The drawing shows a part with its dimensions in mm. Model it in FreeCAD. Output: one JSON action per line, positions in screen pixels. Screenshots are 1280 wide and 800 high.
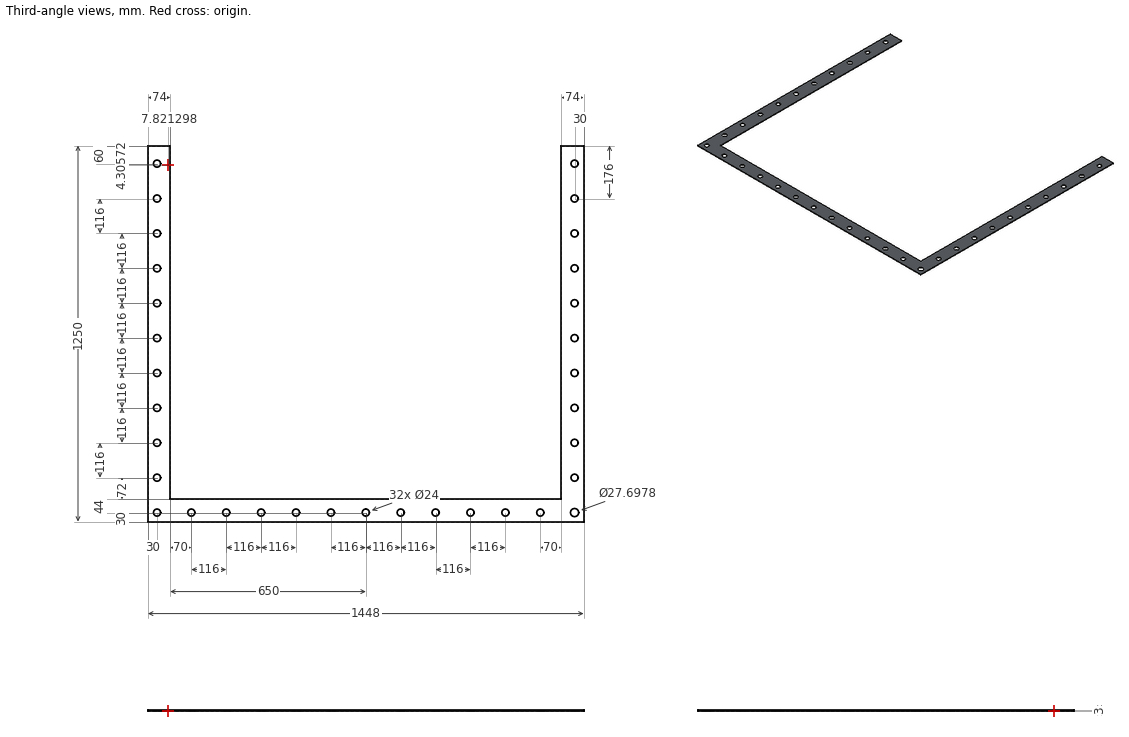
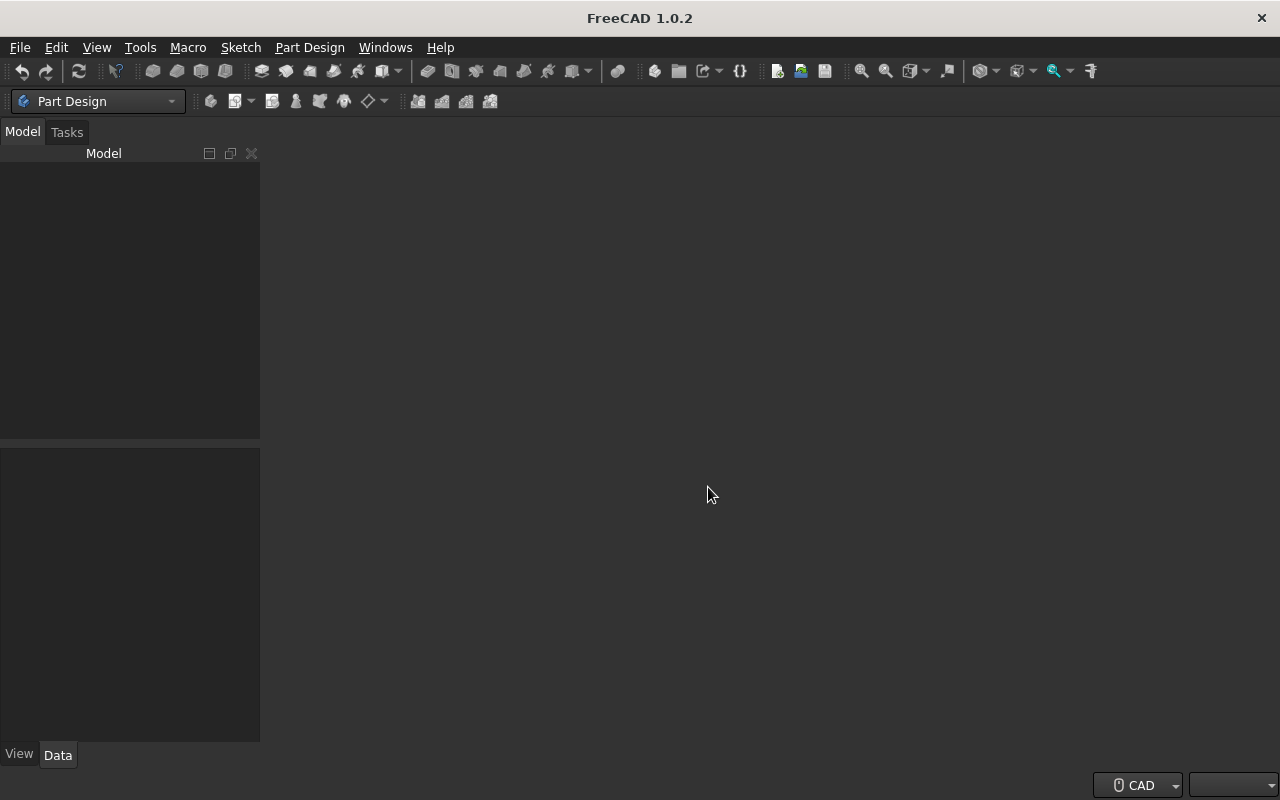
{"action": "left_click", "coordinate": [778, 72]}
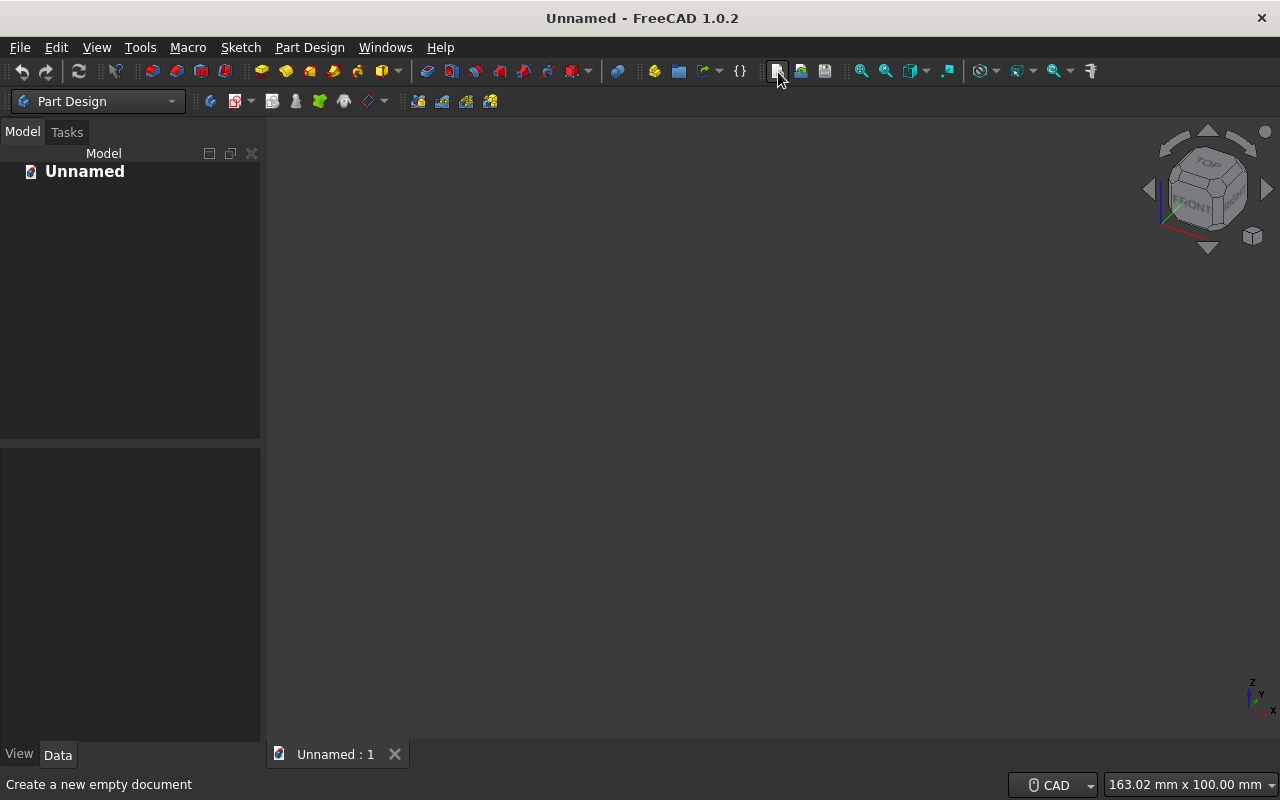
{"action": "left_click", "coordinate": [236, 102]}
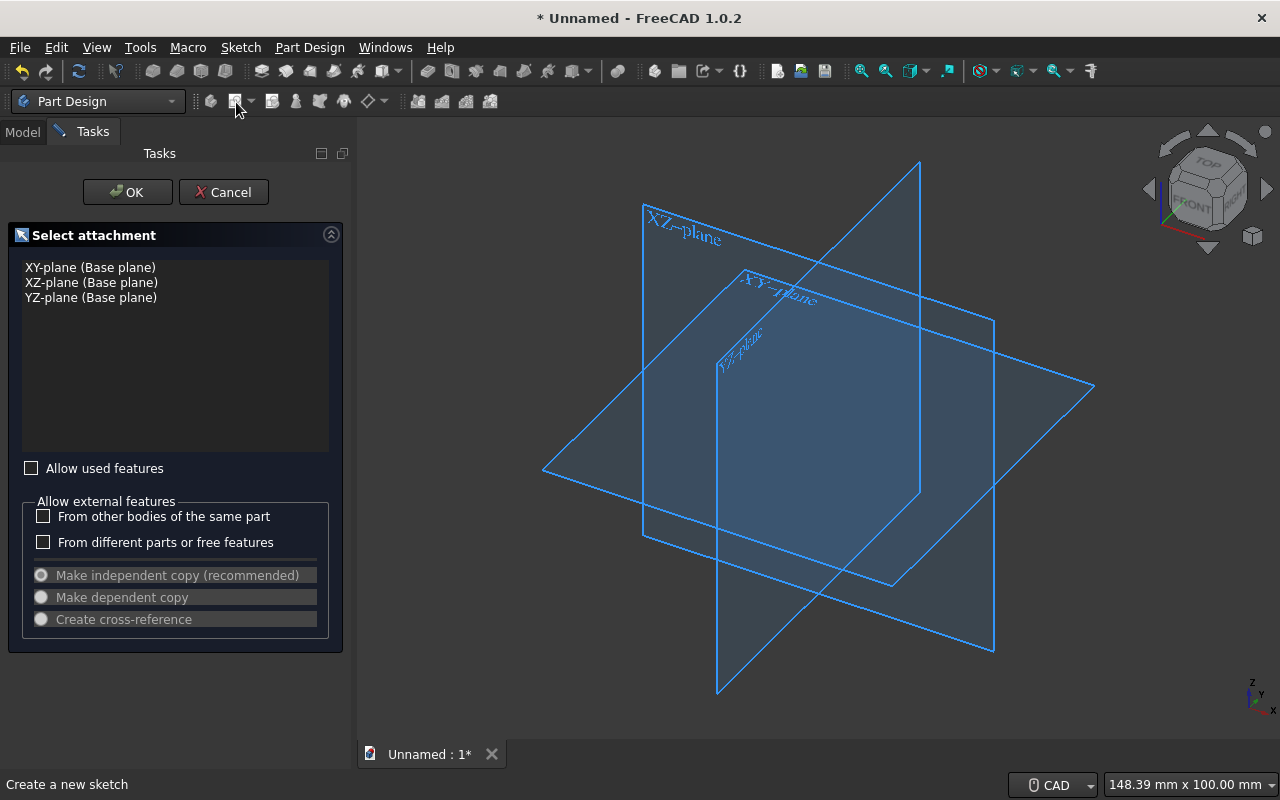
{"action": "left_click", "coordinate": [82, 268]}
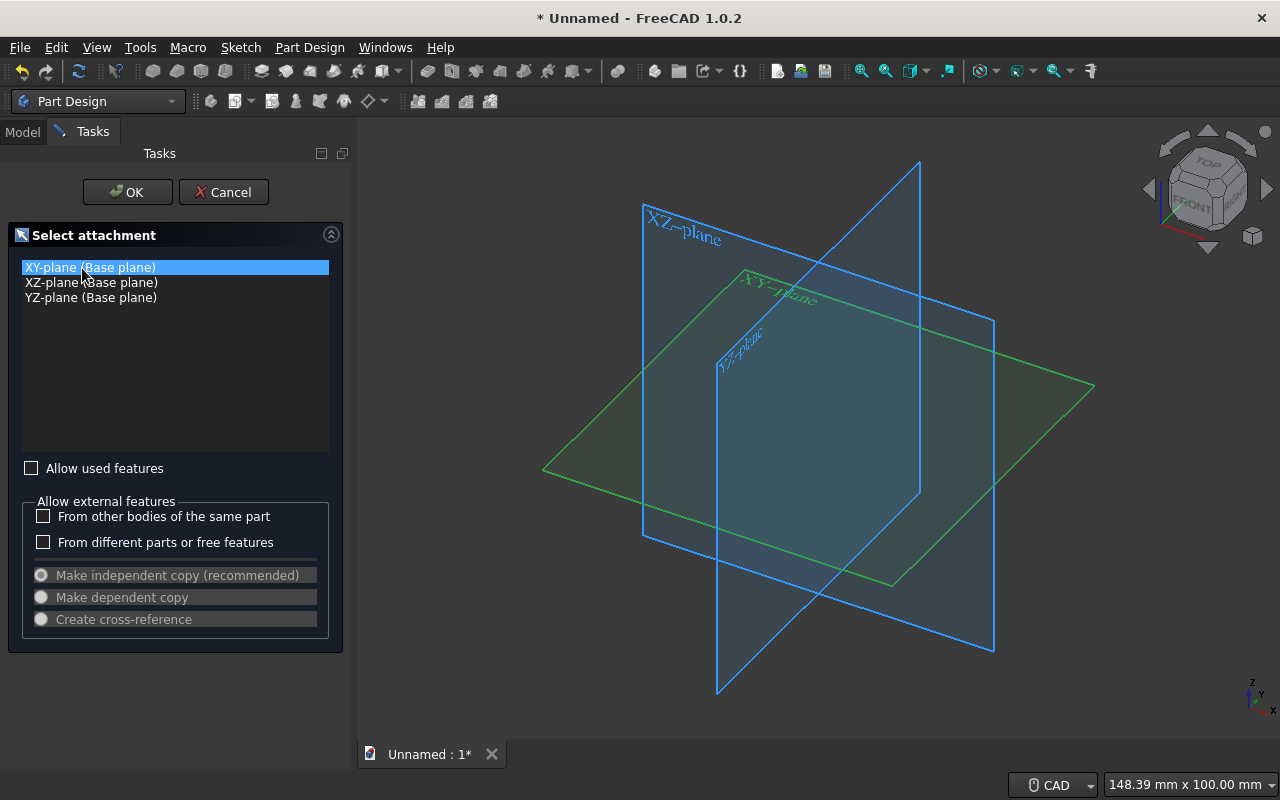
{"action": "left_click", "coordinate": [128, 192]}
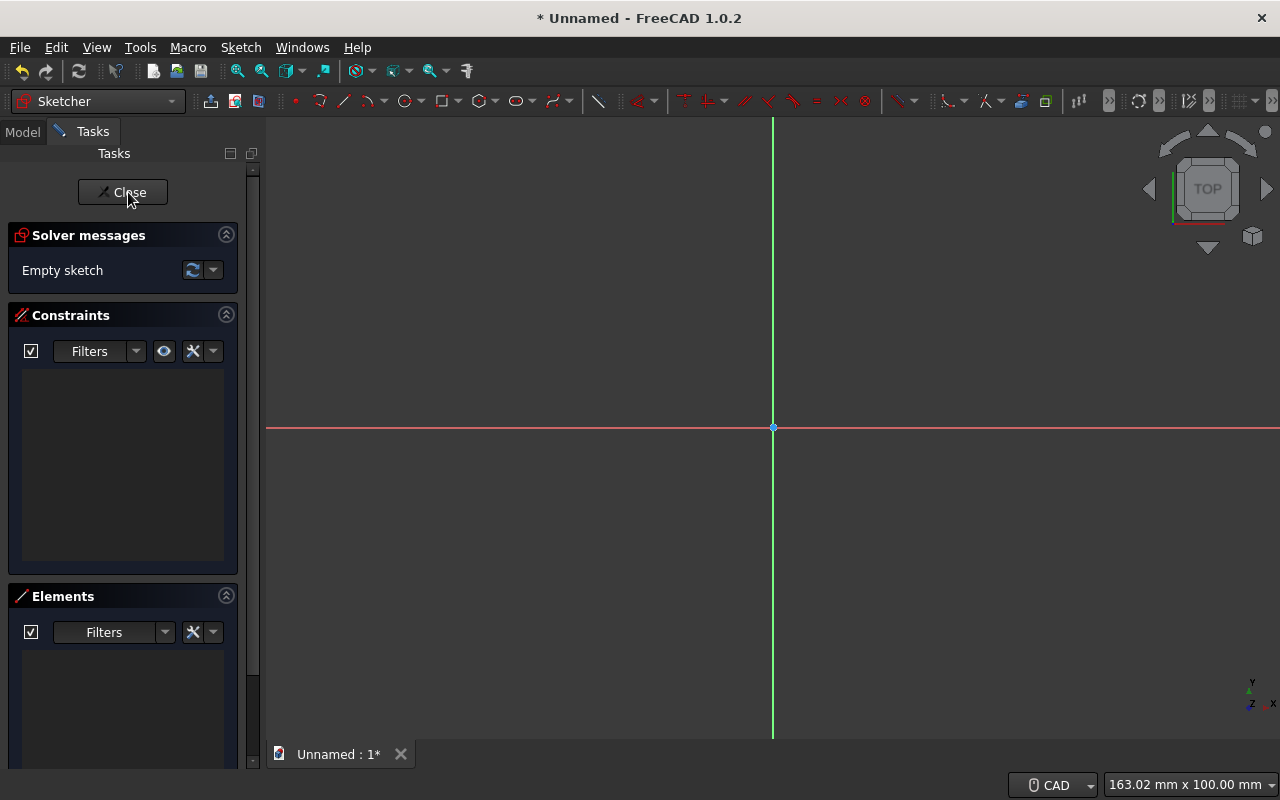
{"action": "scroll", "coordinate": [487, 245], "scroll_direction": "down", "scroll_amount": 15}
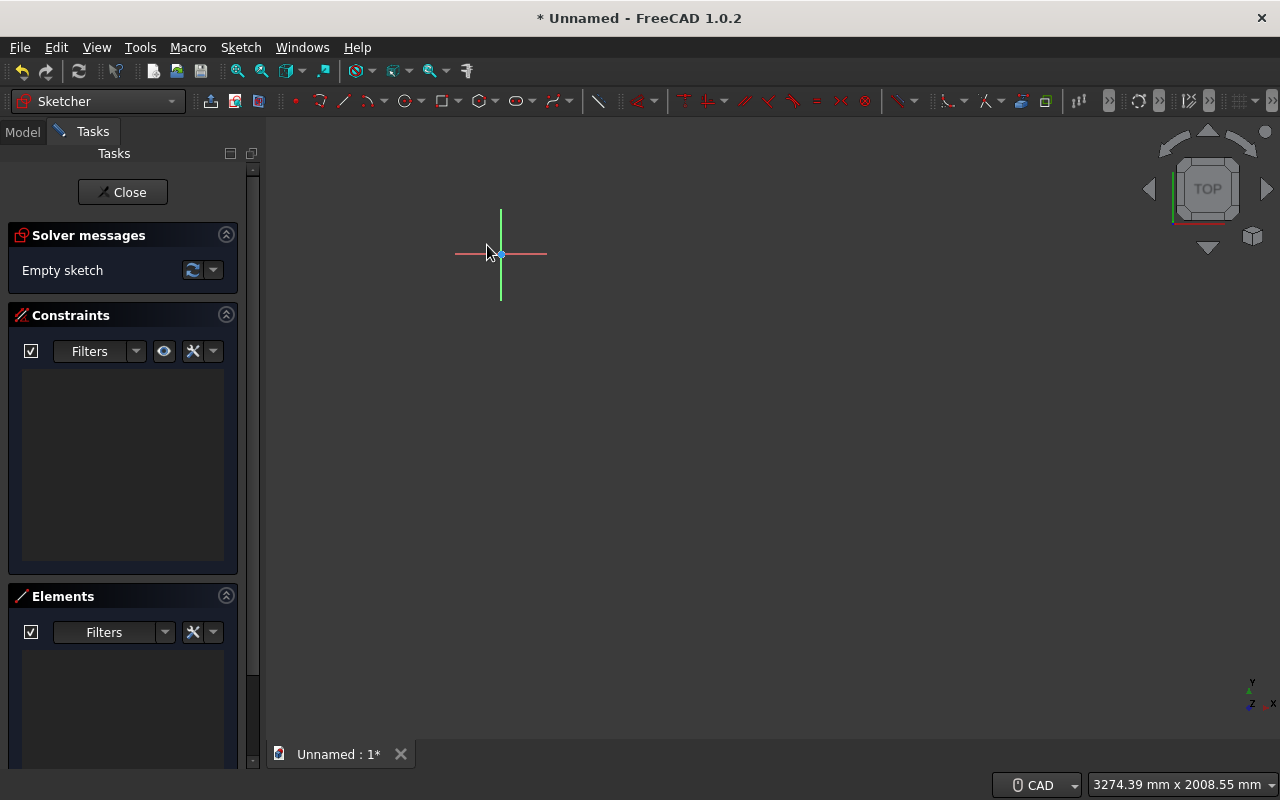
{"action": "left_click", "coordinate": [320, 102]}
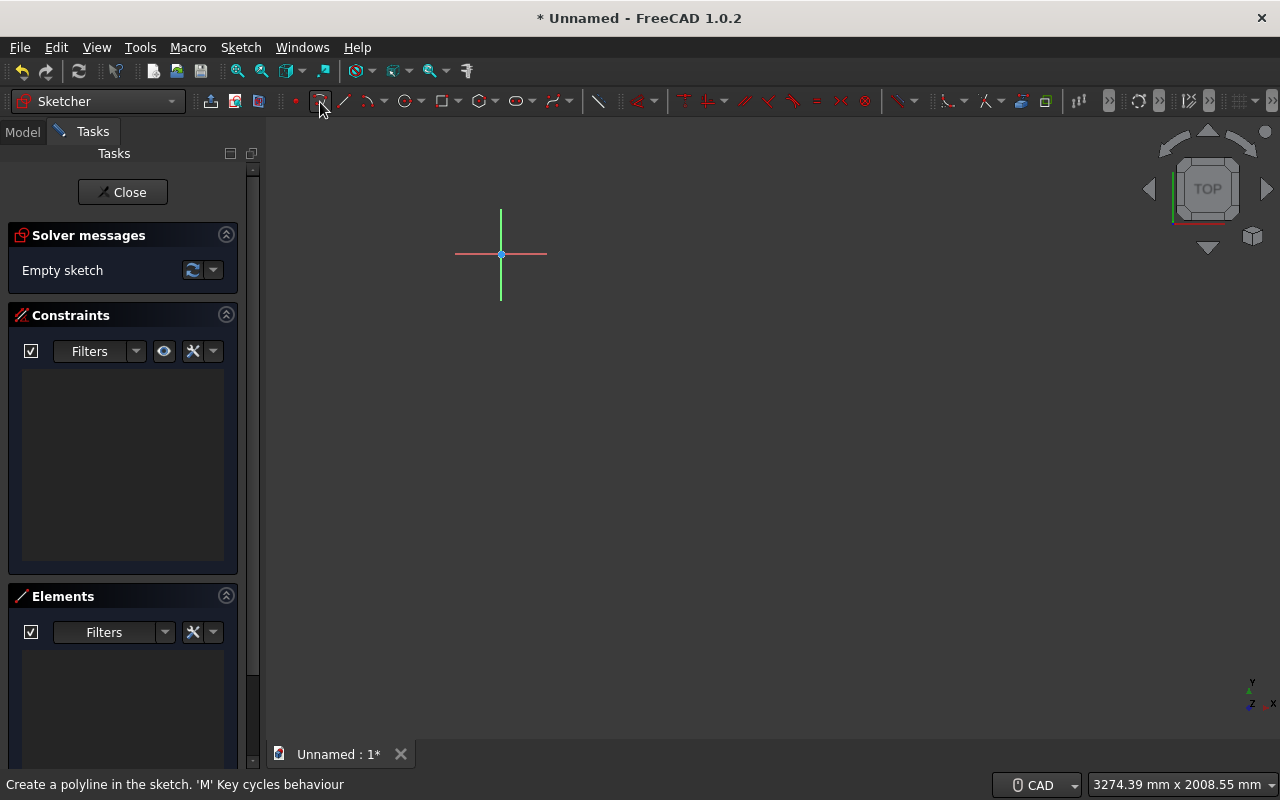
{"action": "scroll", "coordinate": [504, 234], "scroll_direction": "up", "scroll_amount": 10}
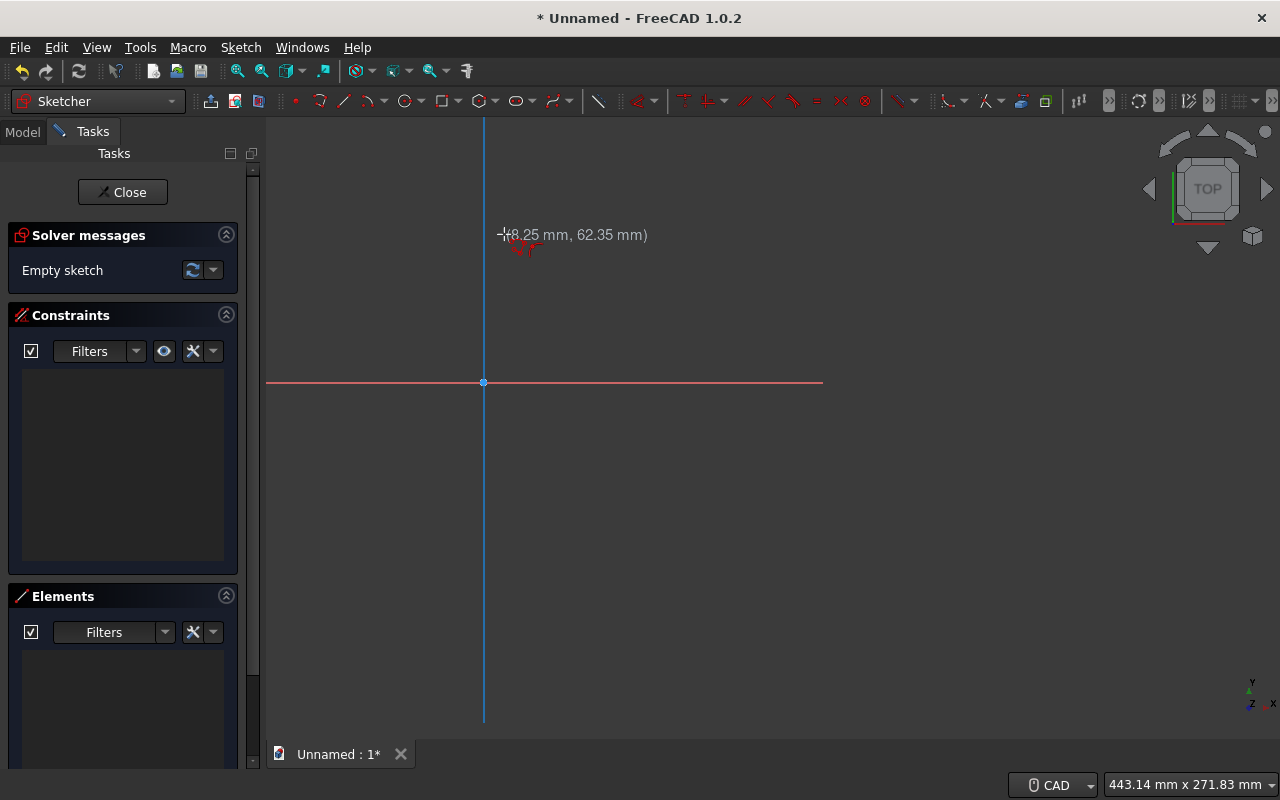
{"action": "left_click", "coordinate": [502, 236]}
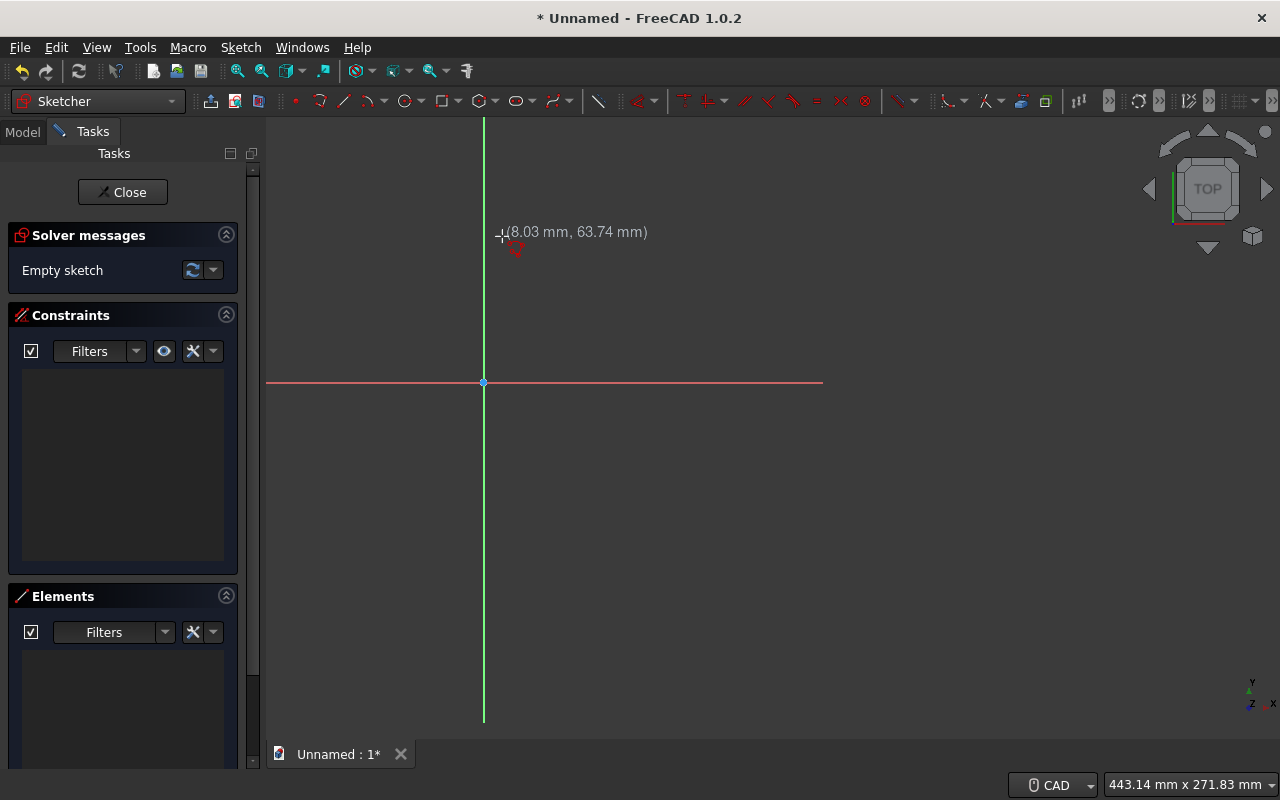
{"action": "scroll", "coordinate": [503, 234], "scroll_direction": "down", "scroll_amount": 10}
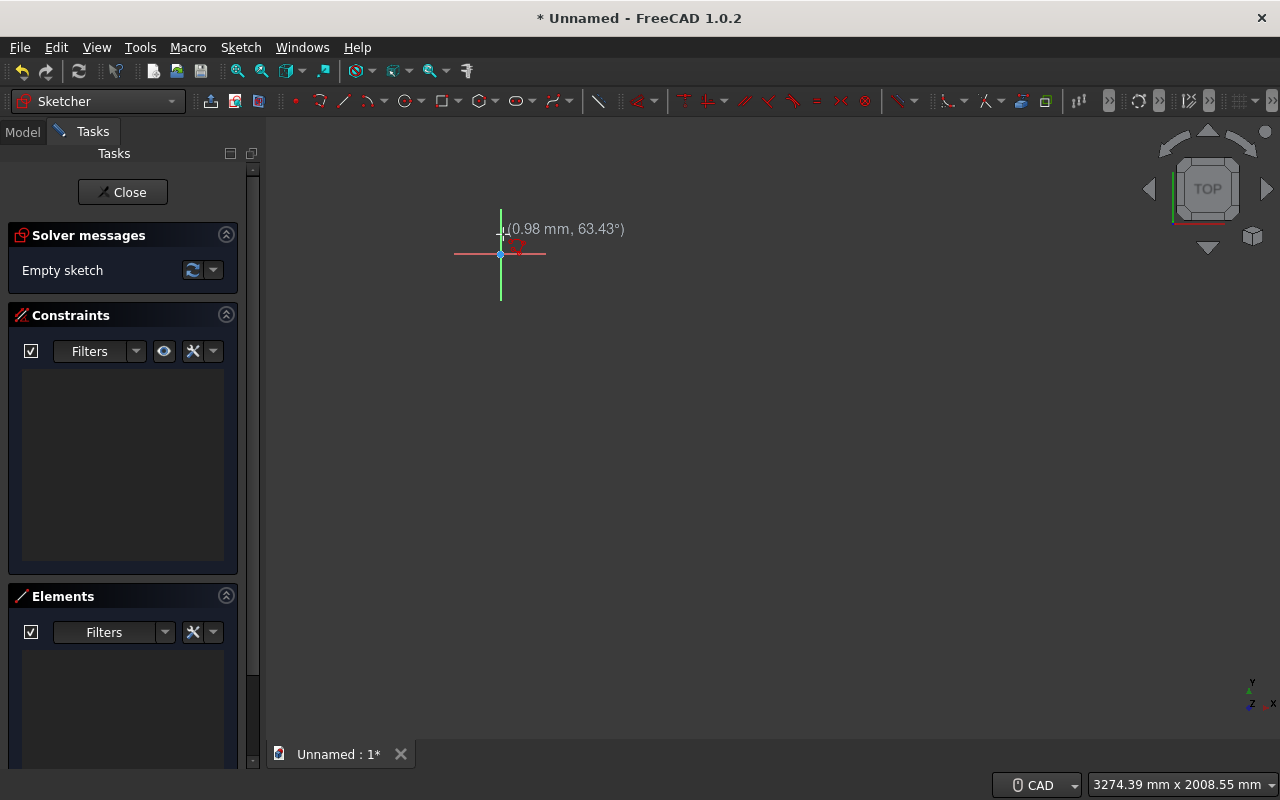
{"action": "left_click", "coordinate": [480, 234]}
{"action": "left_click", "coordinate": [480, 621]}
{"action": "left_click", "coordinate": [928, 621]}
{"action": "left_click", "coordinate": [928, 234]}
{"action": "left_click", "coordinate": [906, 234]}
{"action": "left_click", "coordinate": [906, 599]}